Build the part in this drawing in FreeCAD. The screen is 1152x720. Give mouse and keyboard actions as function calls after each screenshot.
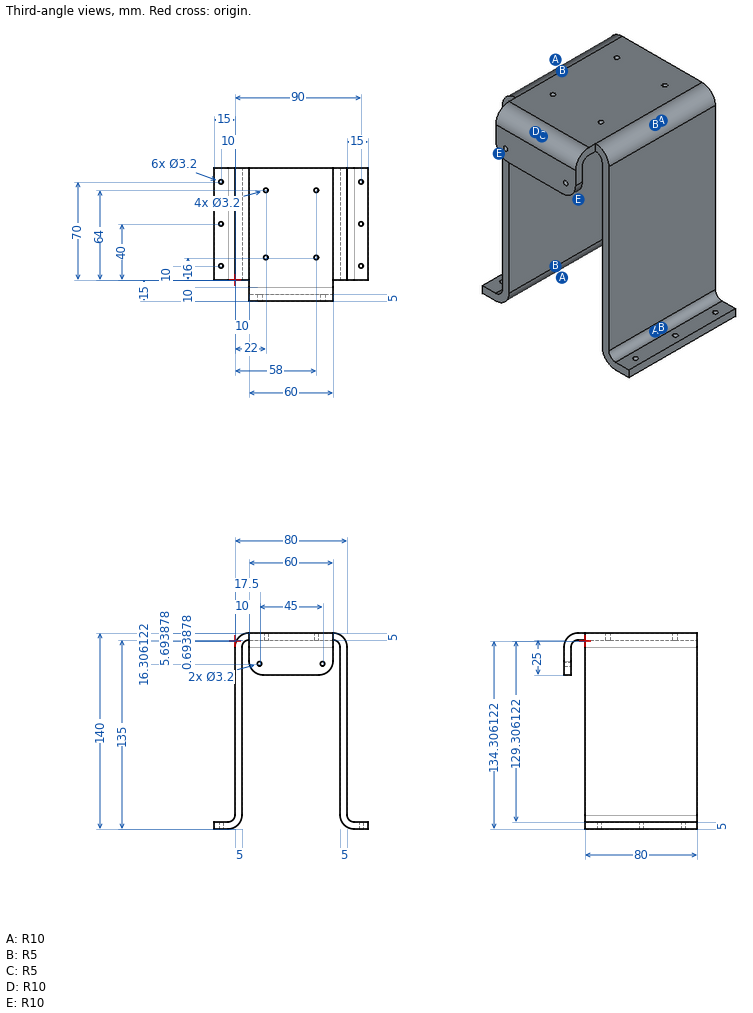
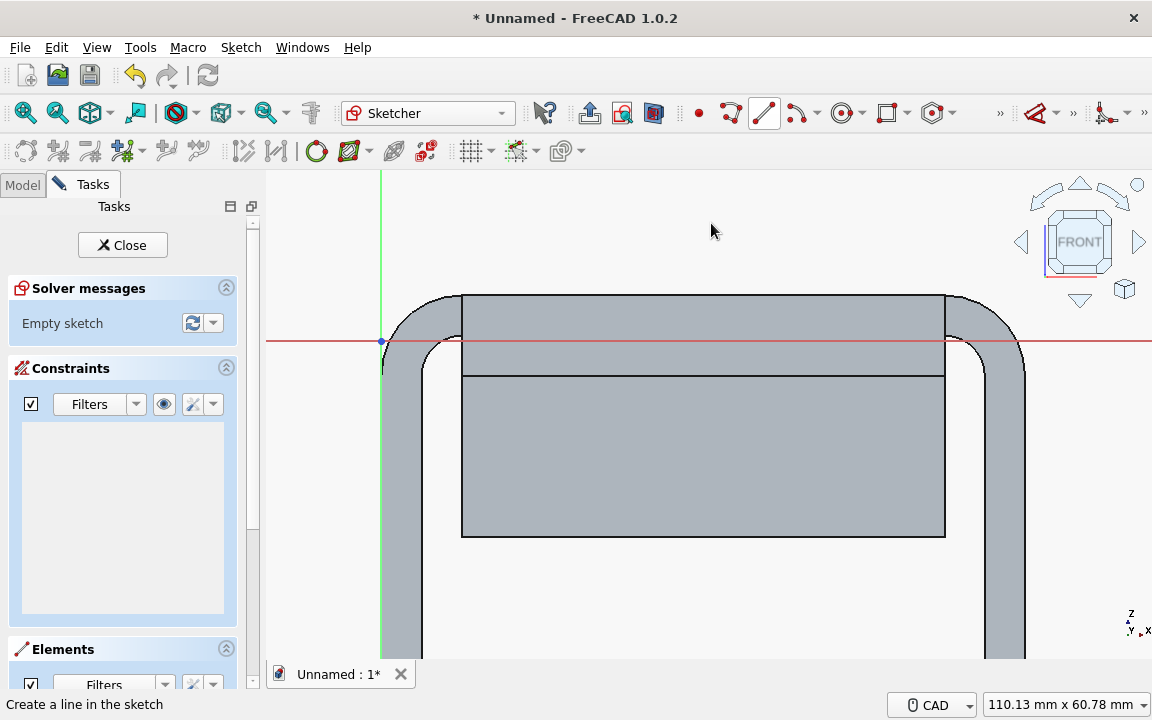
click(842, 114)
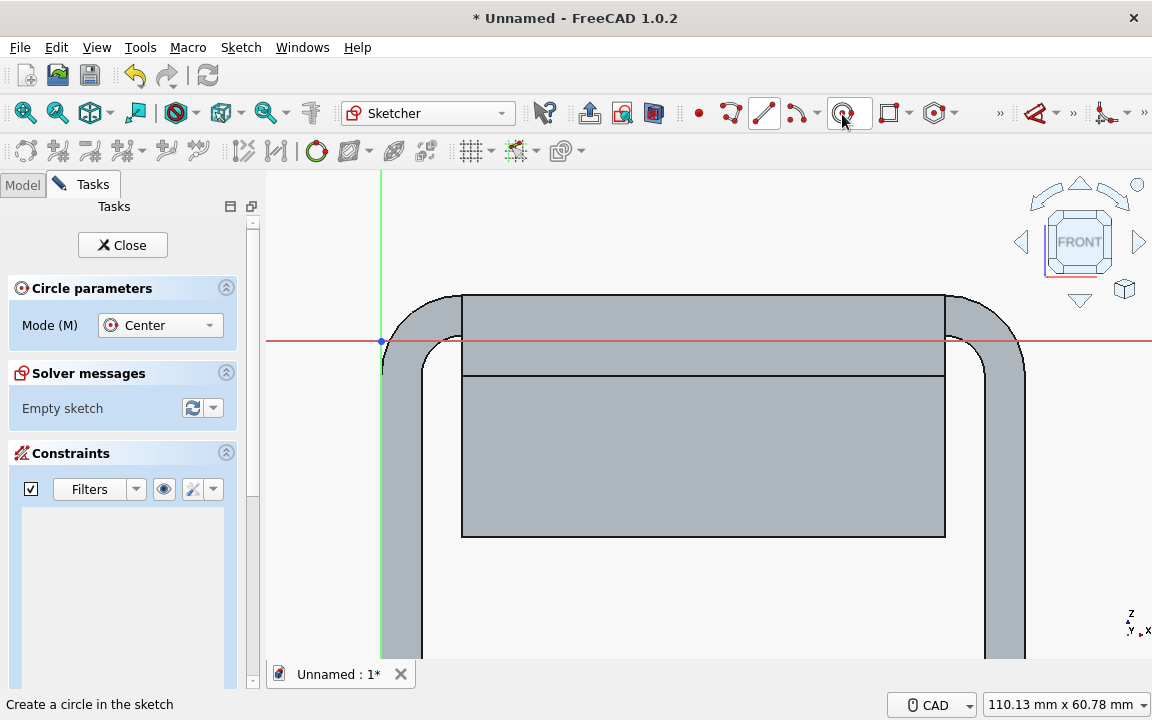
scroll(522, 472, up, 3)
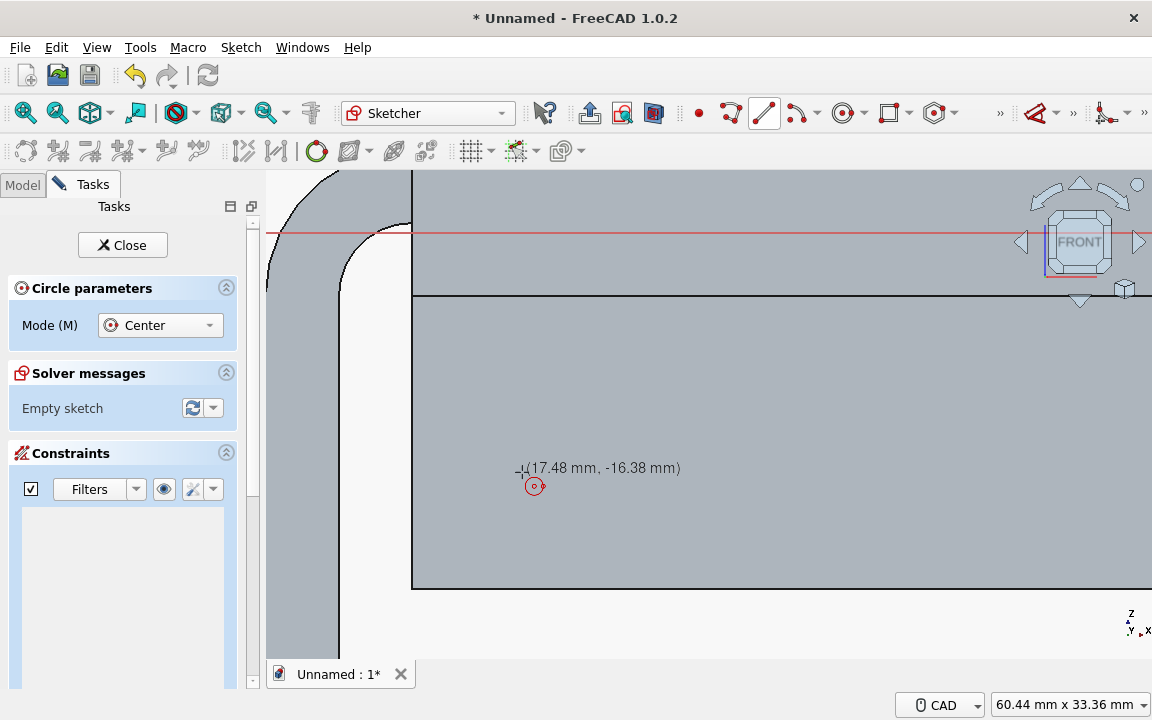
click(522, 472)
move(539, 456)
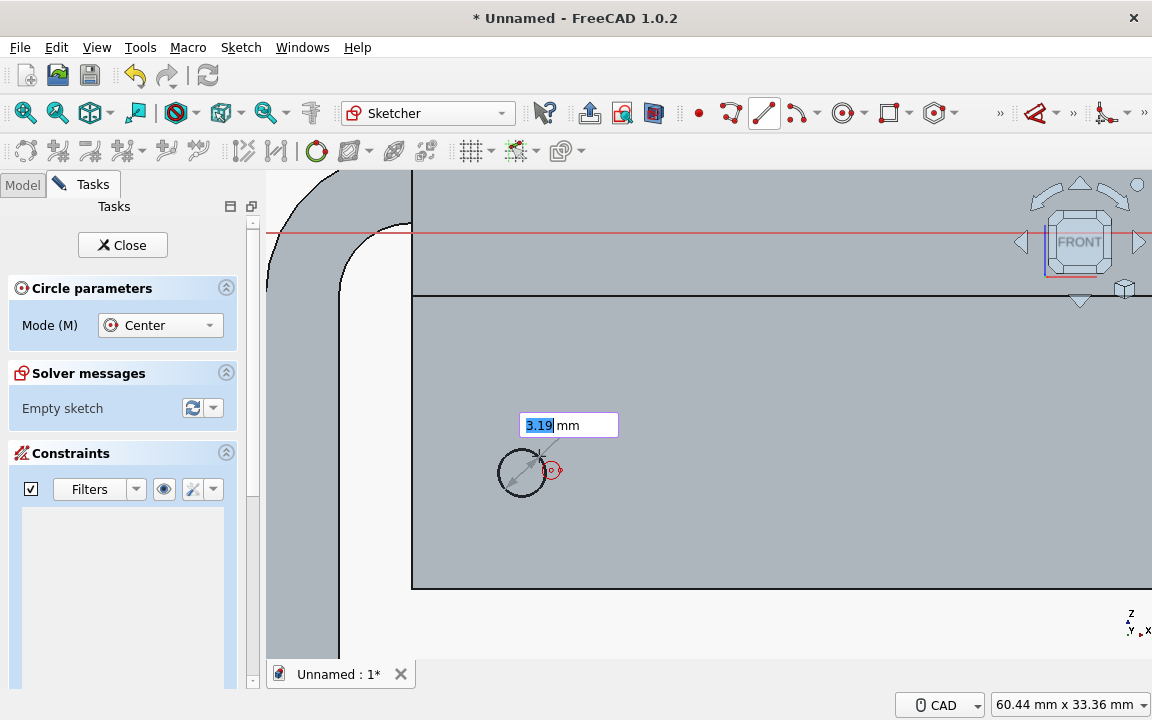
text(3.2)
key(Return)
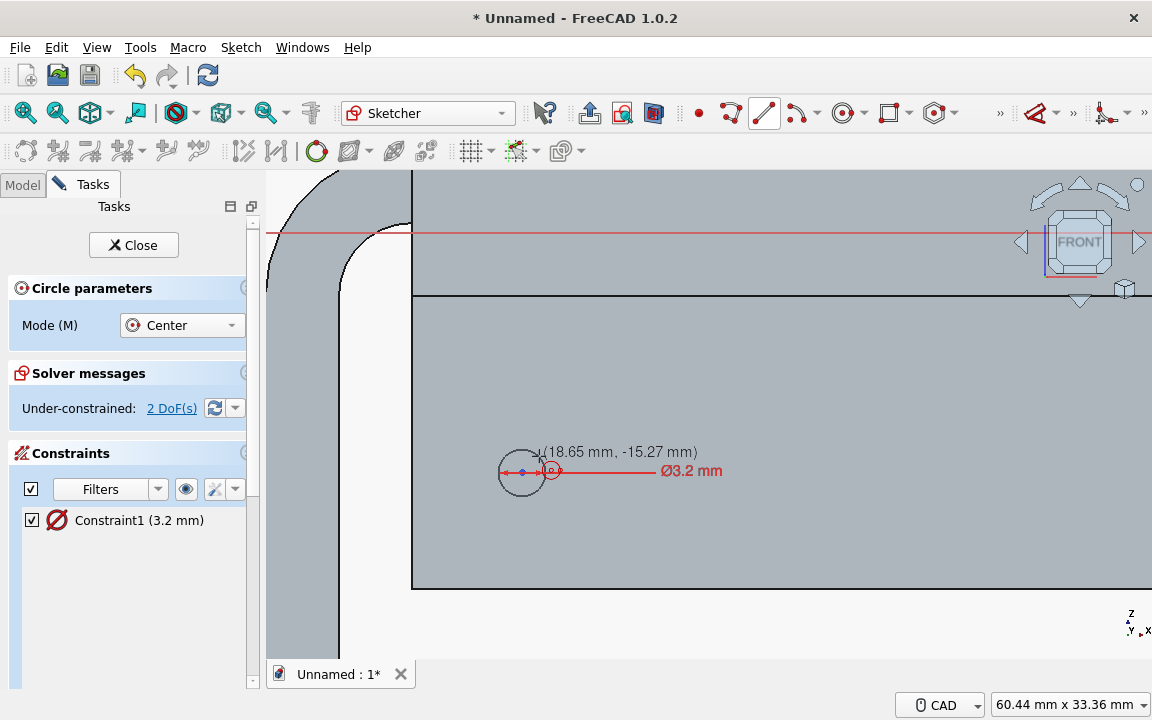
scroll(525, 475, down, 3)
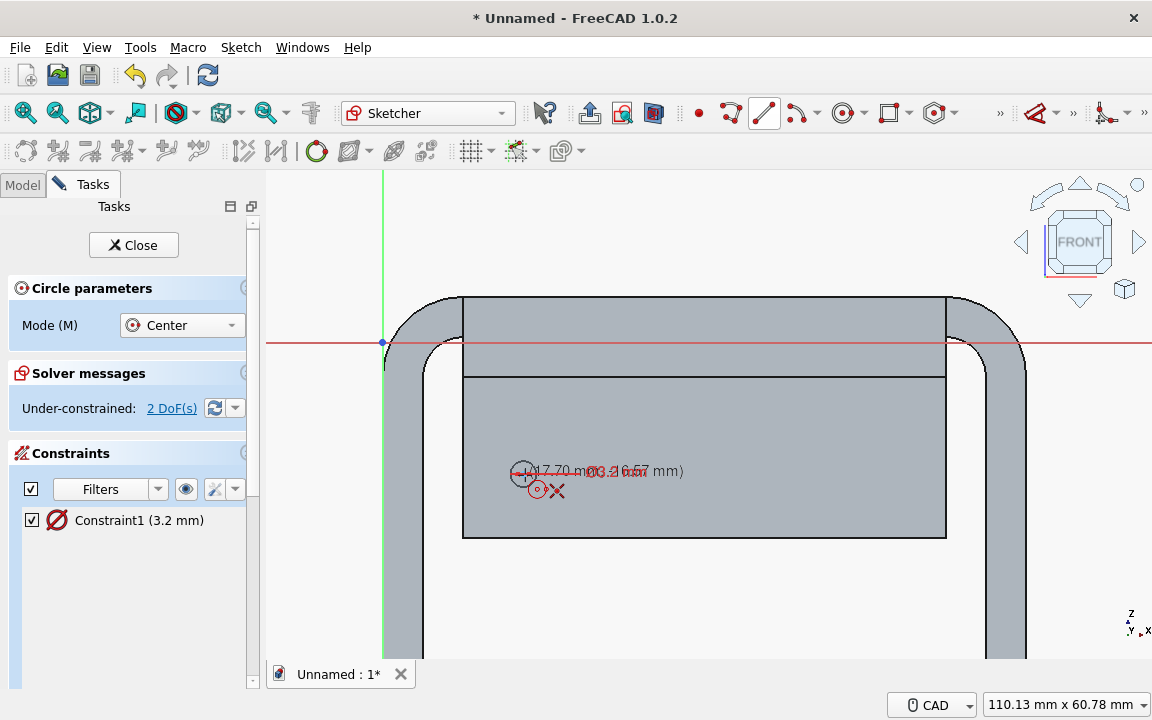
scroll(886, 474, up, 3)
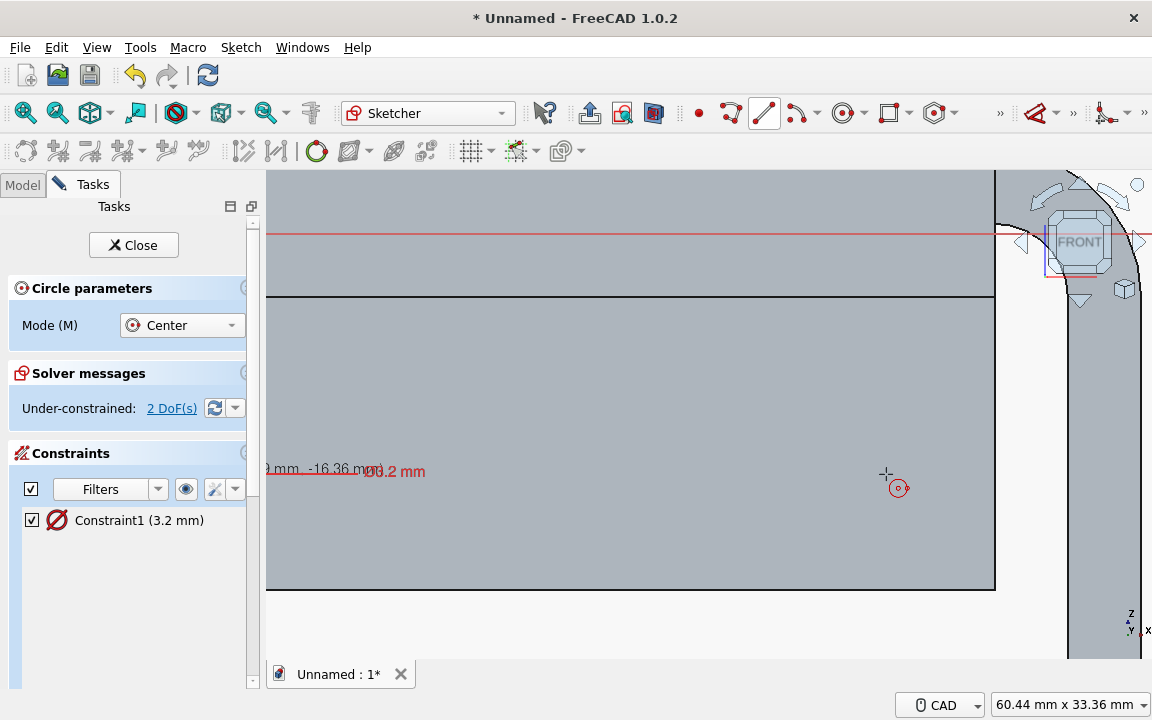
click(885, 473)
move(901, 456)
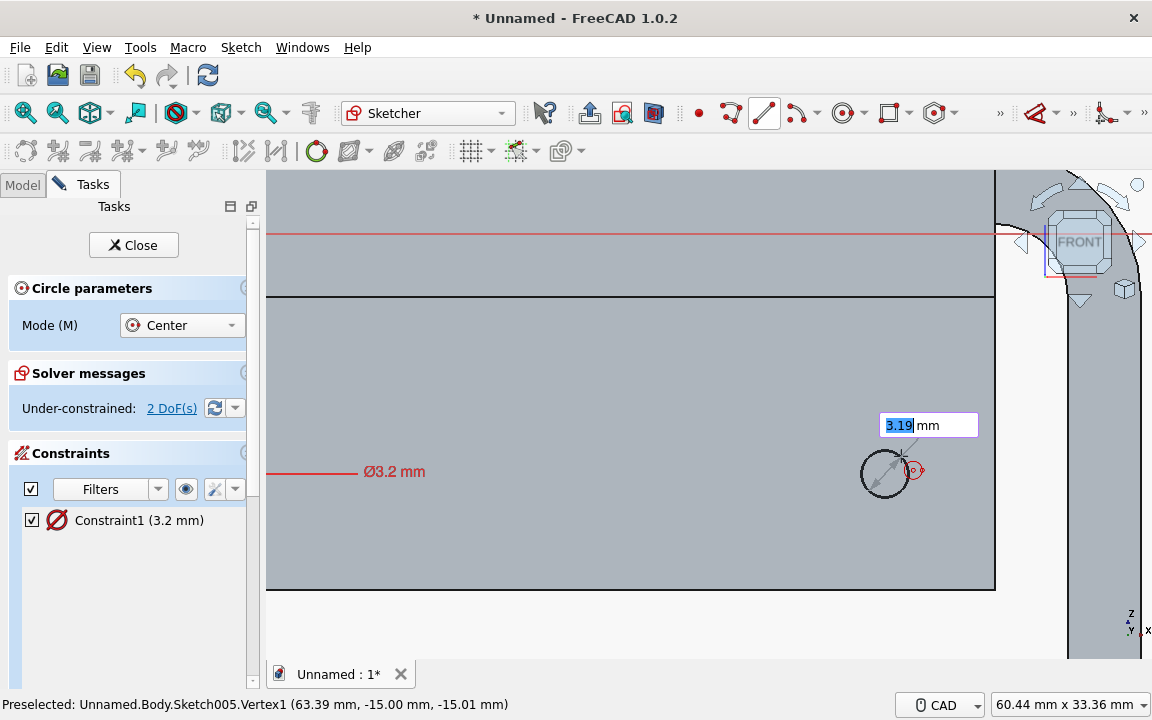
text(3.2)
key(Return)
key(Escape)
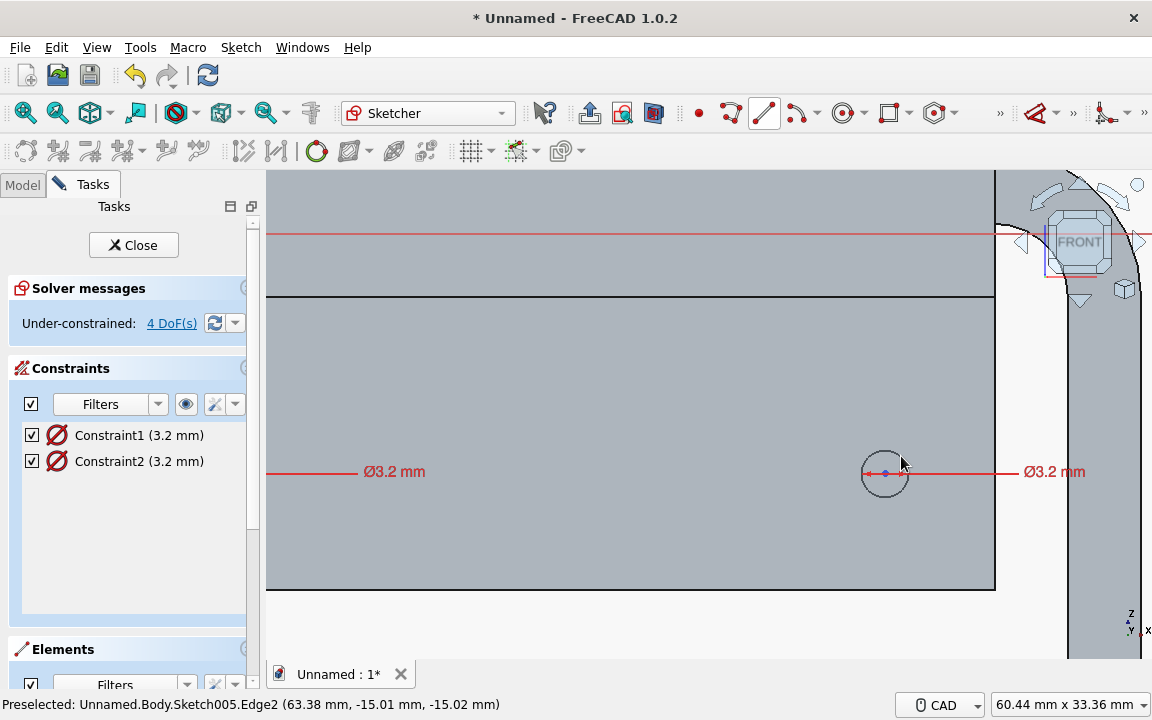
click(1036, 114)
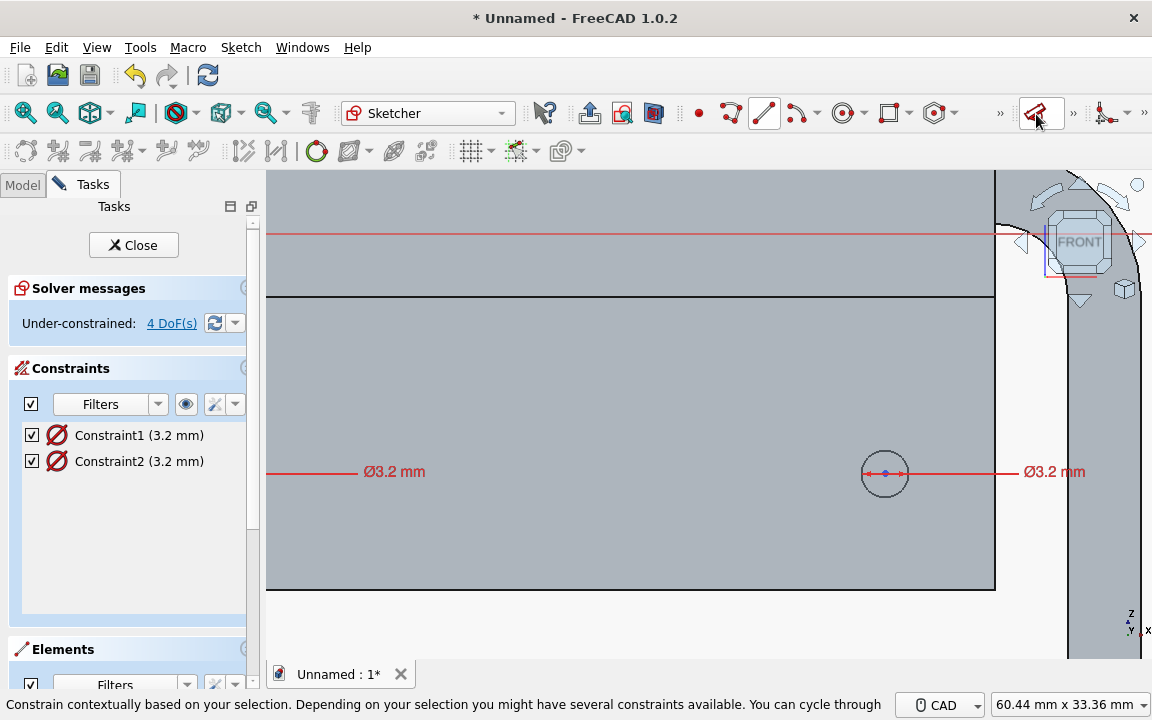
scroll(887, 474, down, 3)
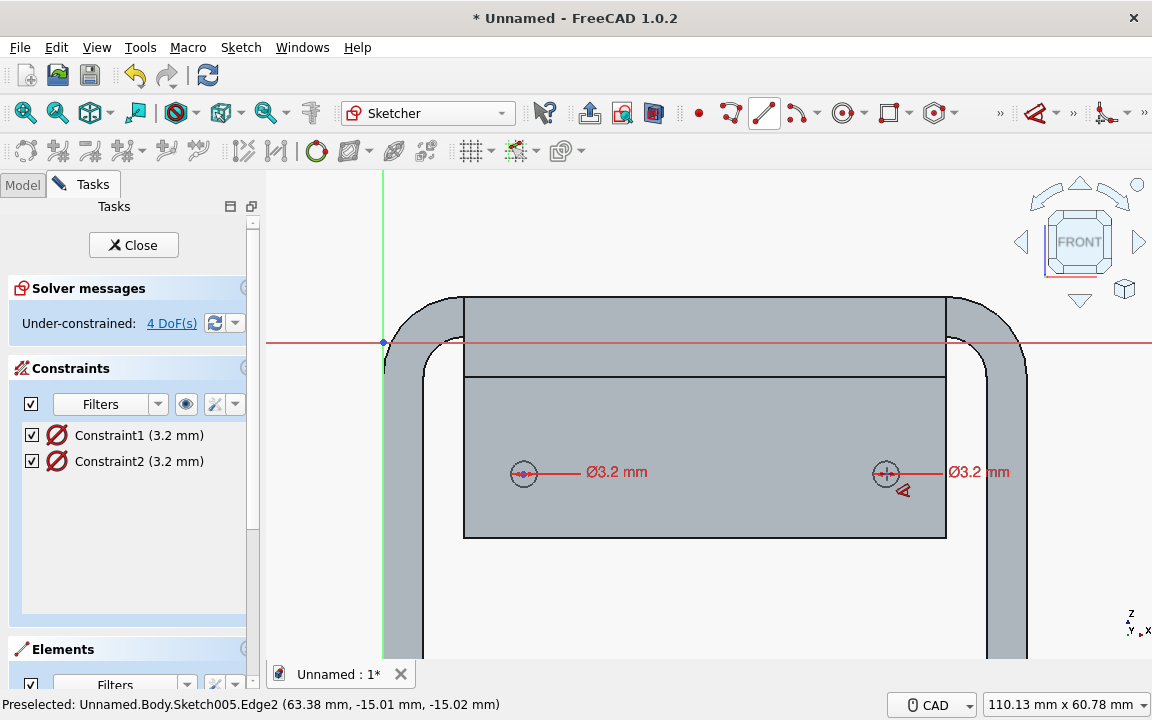
click(524, 474)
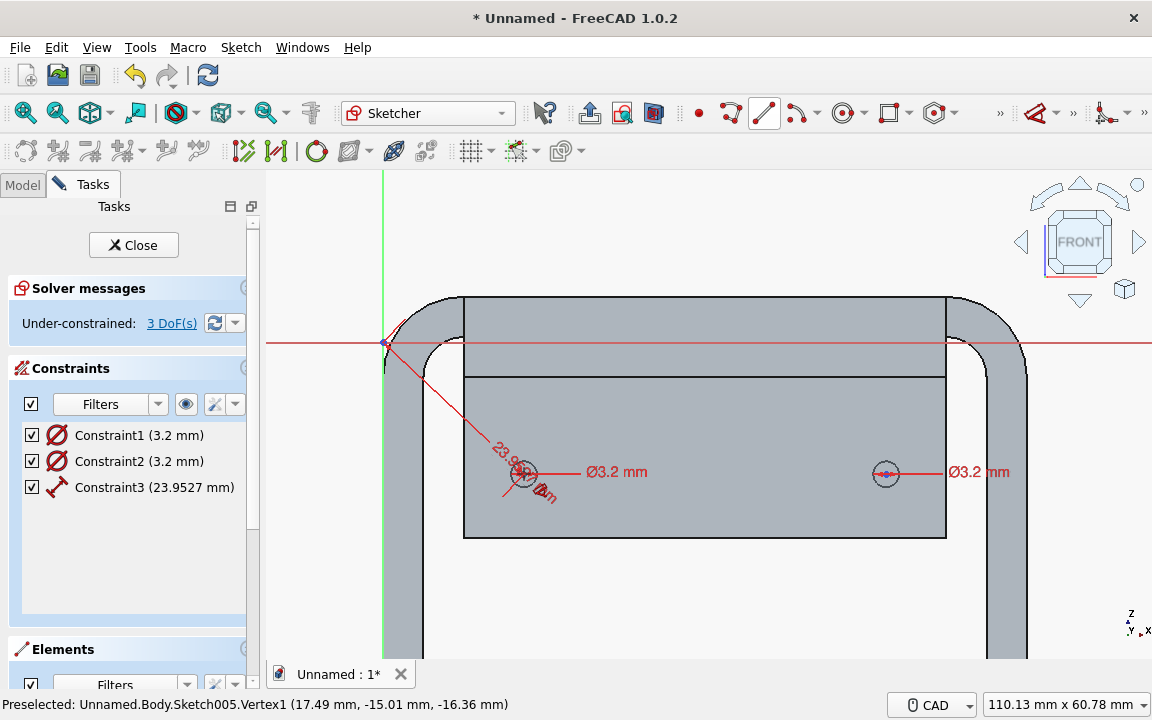
click(886, 474)
click(705, 508)